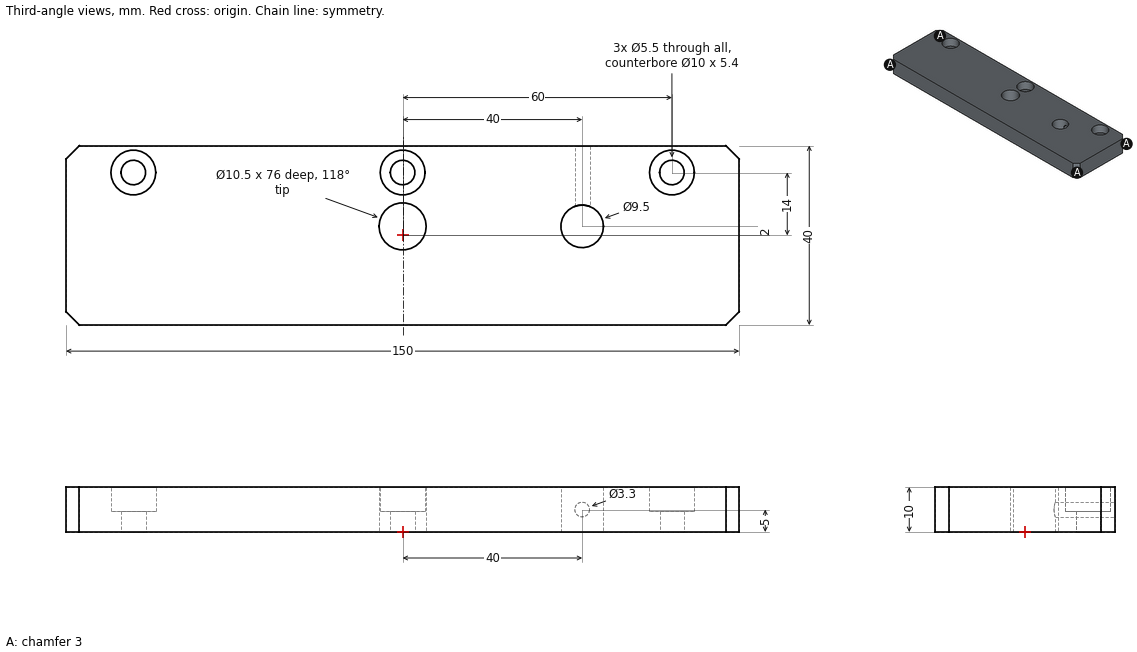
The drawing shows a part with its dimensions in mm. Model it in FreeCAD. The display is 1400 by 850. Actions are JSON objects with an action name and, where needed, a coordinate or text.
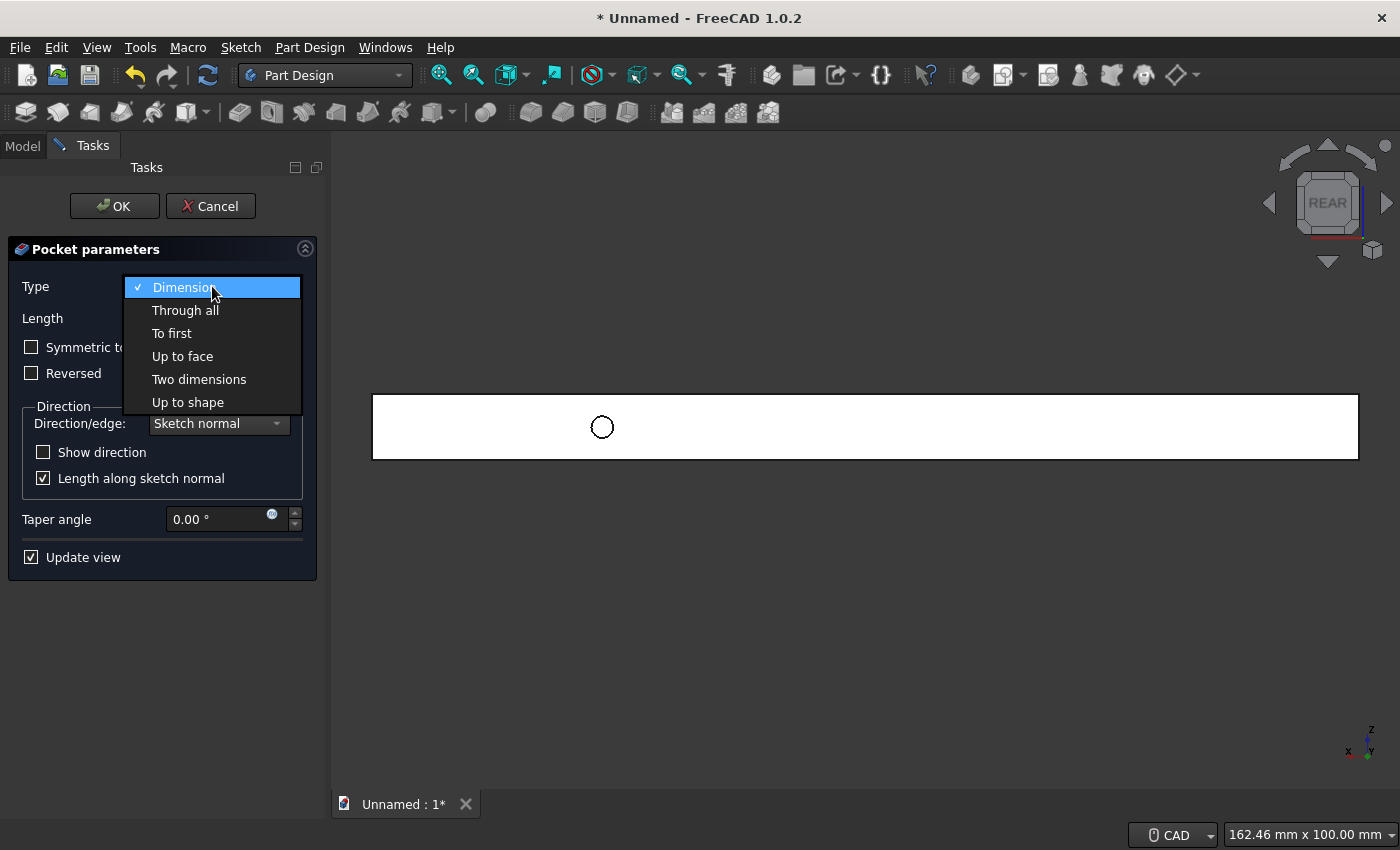
{"action": "left_click", "coordinate": [212, 334]}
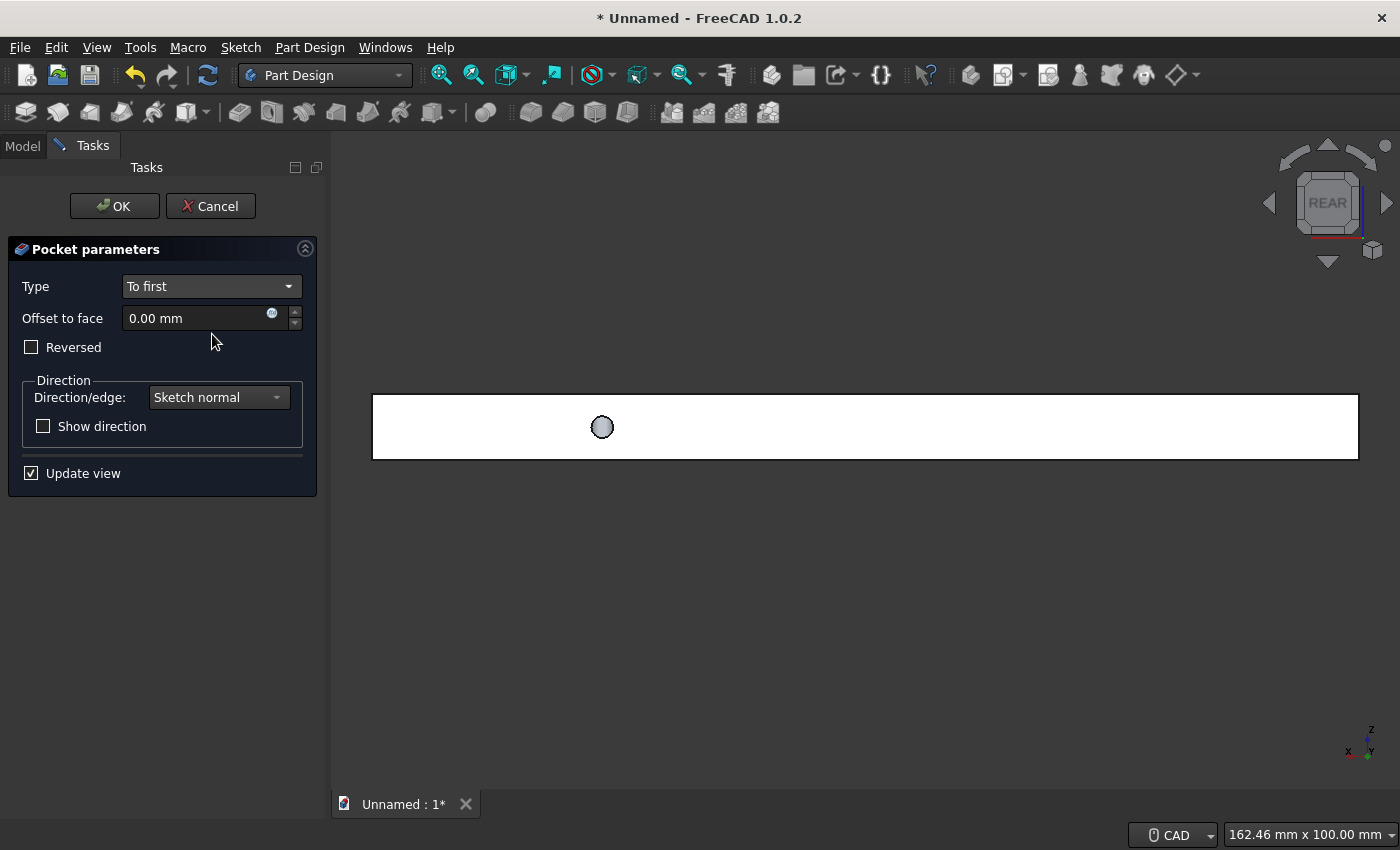
{"action": "left_click", "coordinate": [115, 206]}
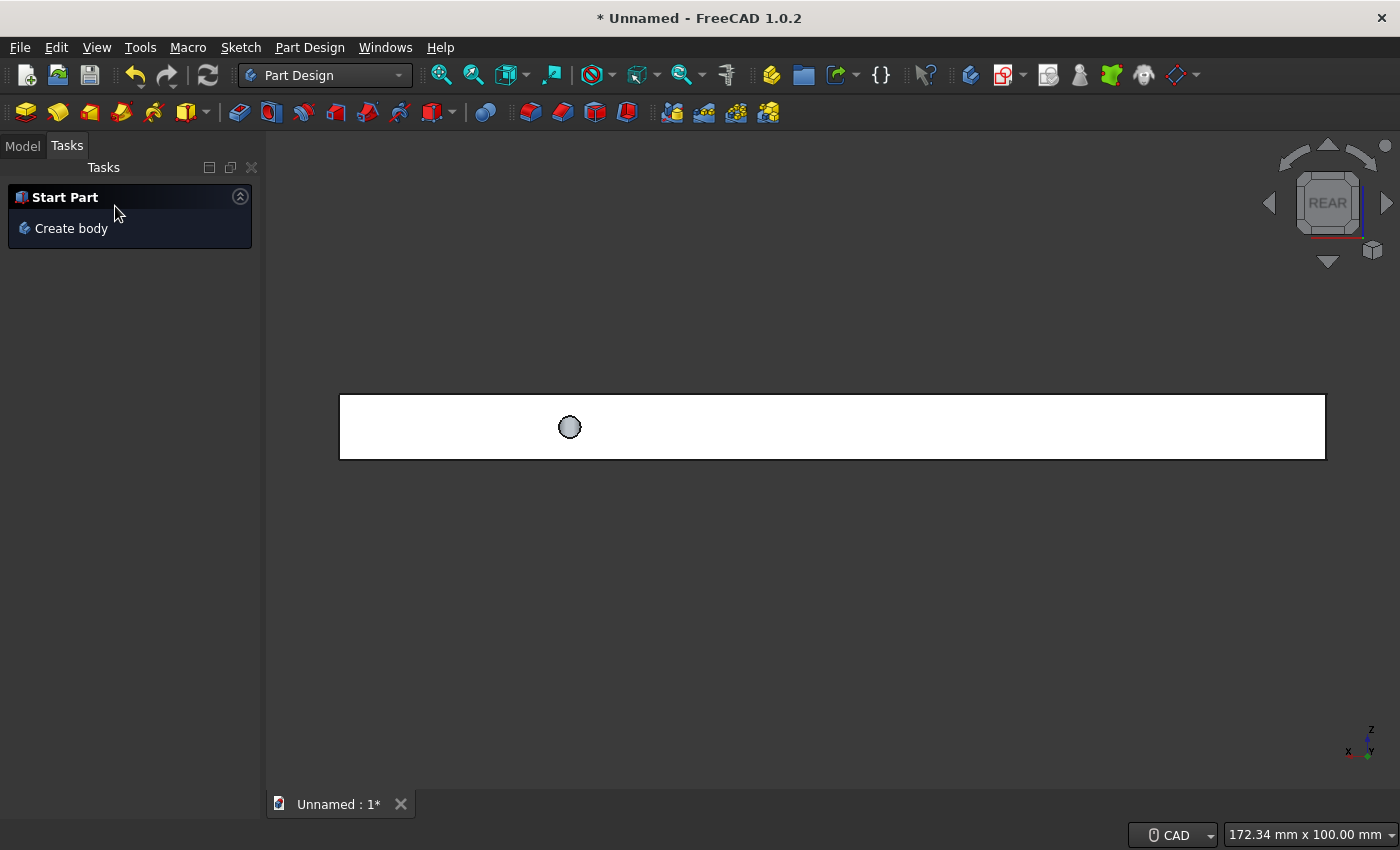
{"action": "left_click", "coordinate": [1327, 426]}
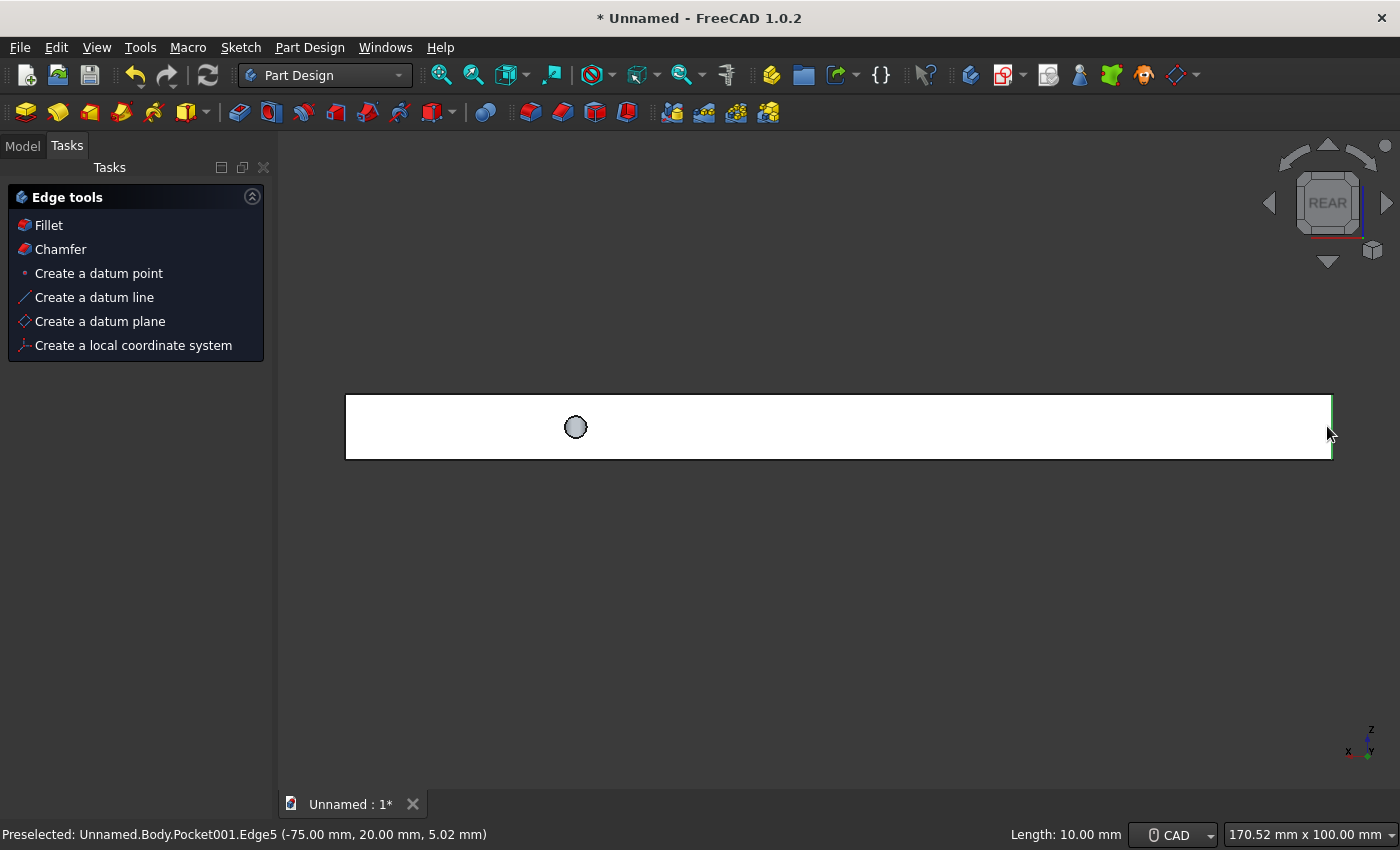
{"action": "key", "text": "0"}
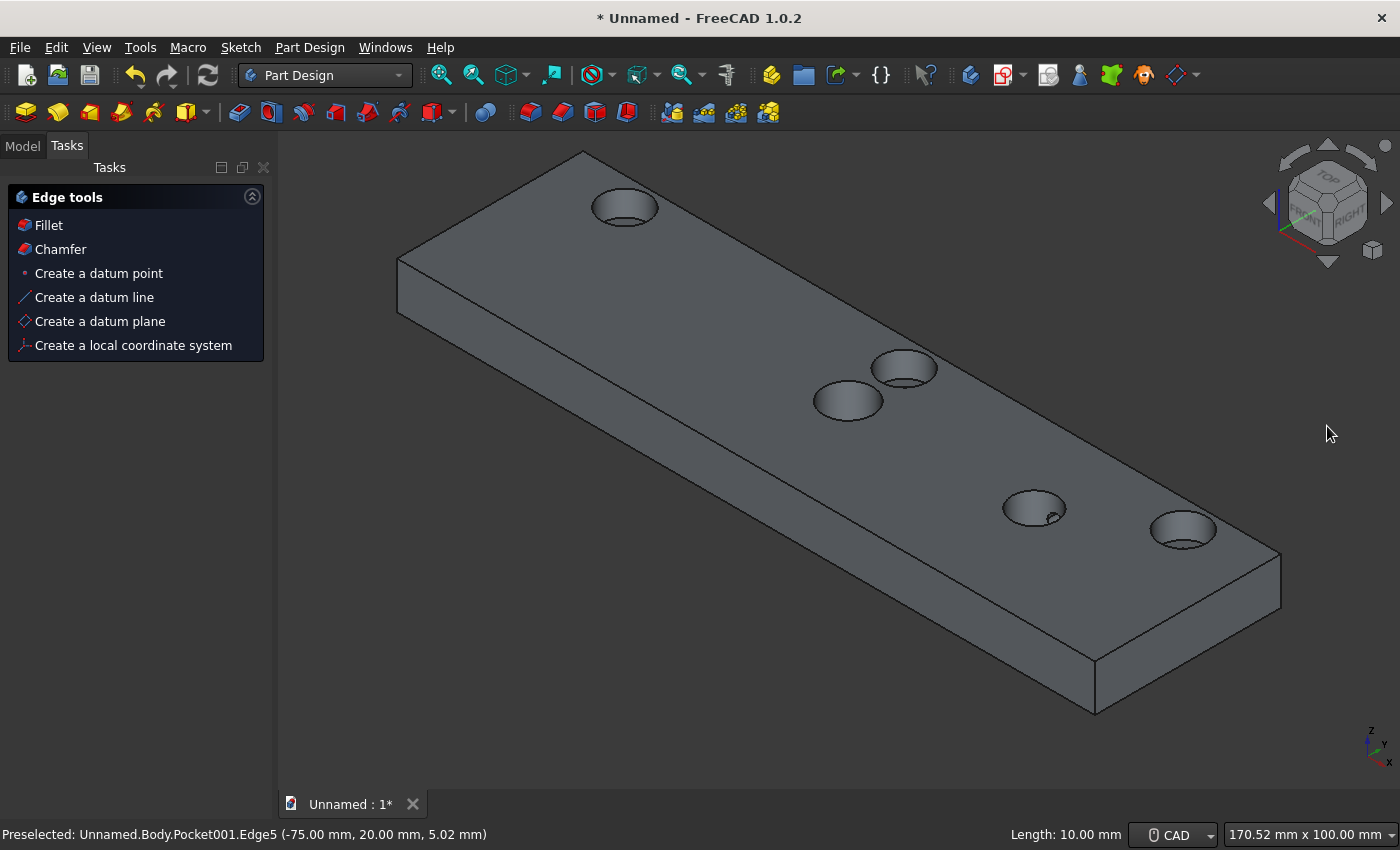
{"action": "left_click", "coordinate": [1095, 687], "text": "ctrl"}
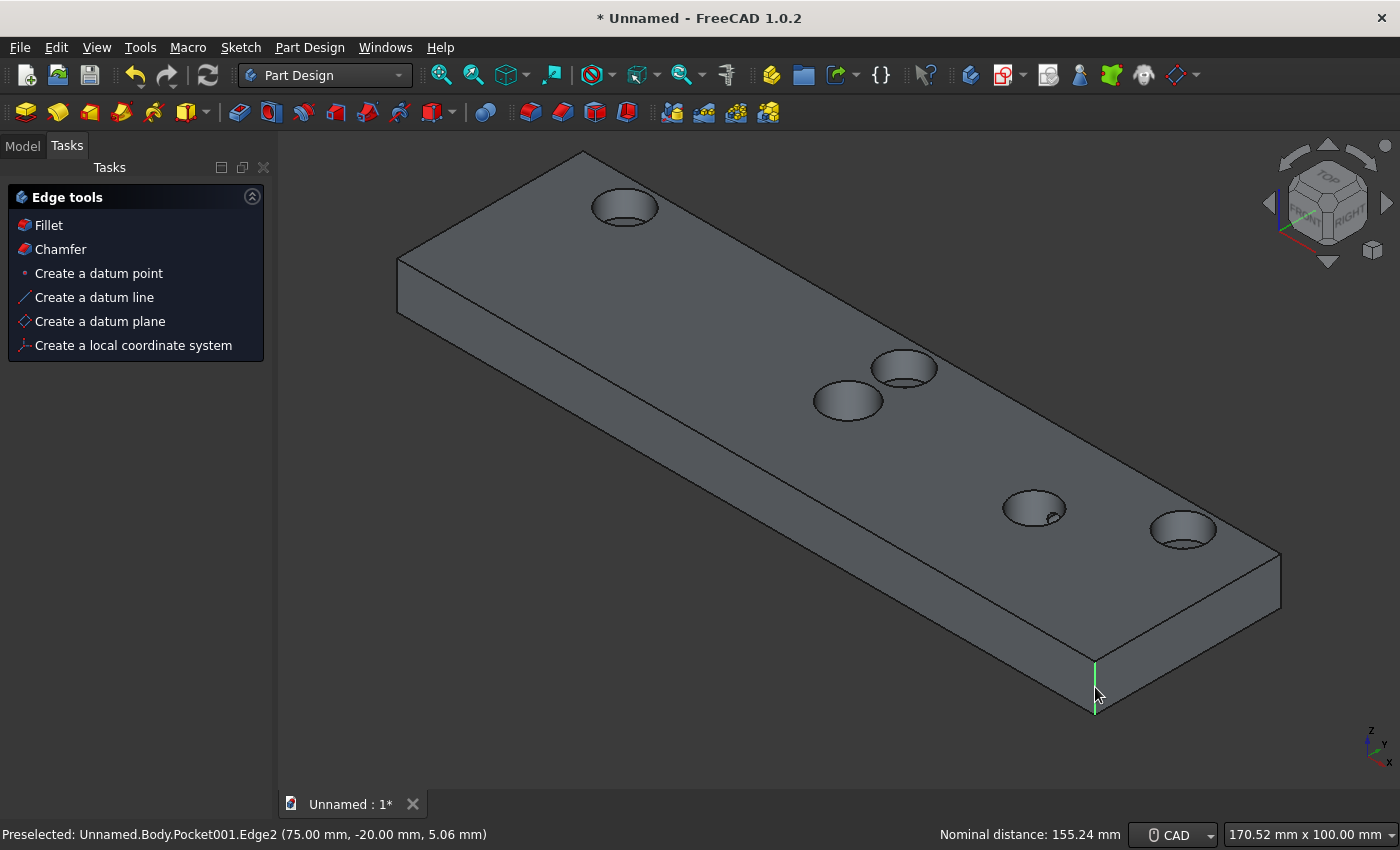
{"action": "key", "text": "2"}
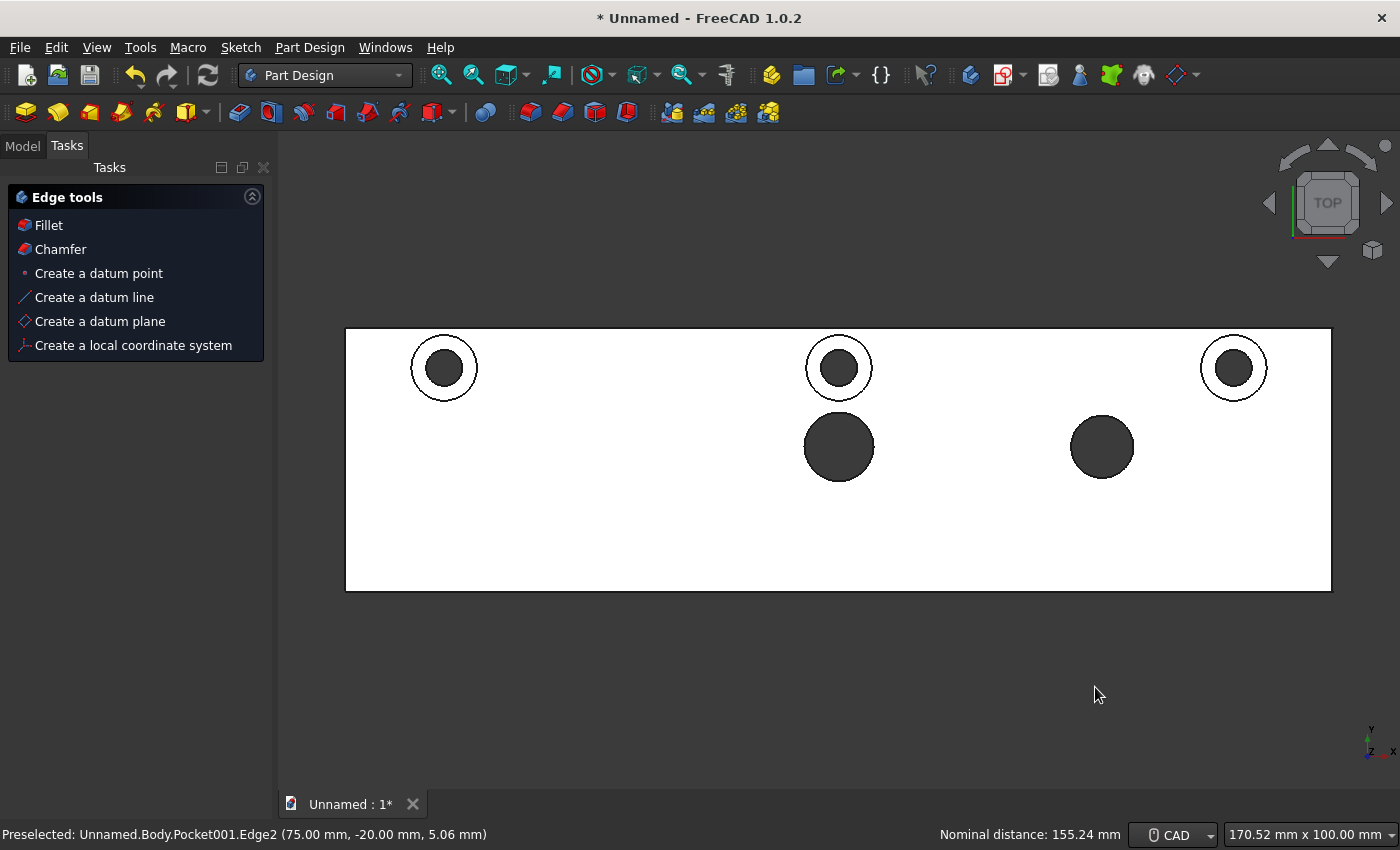
{"action": "key", "text": "1"}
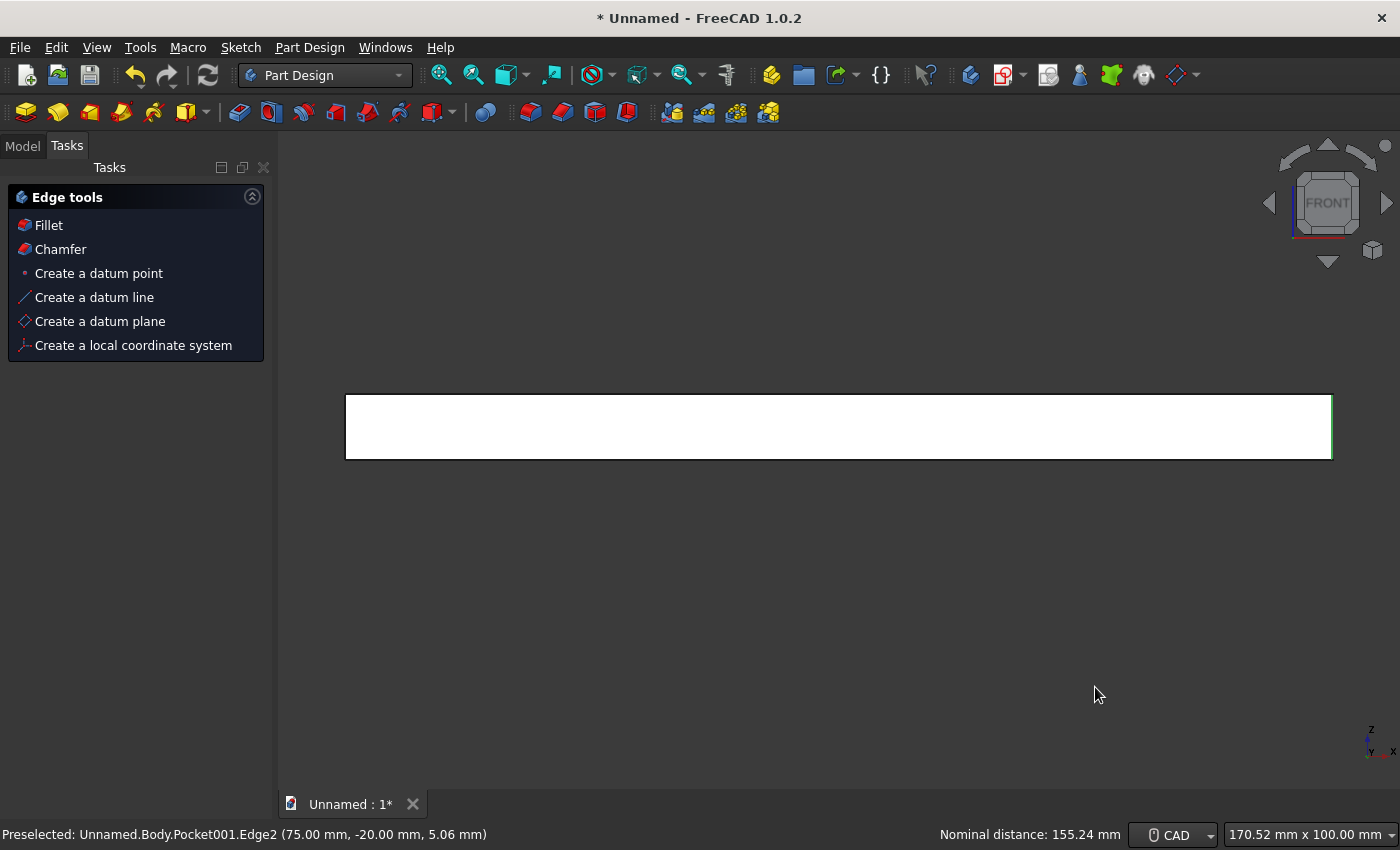
{"action": "left_click", "coordinate": [345, 426], "text": "ctrl"}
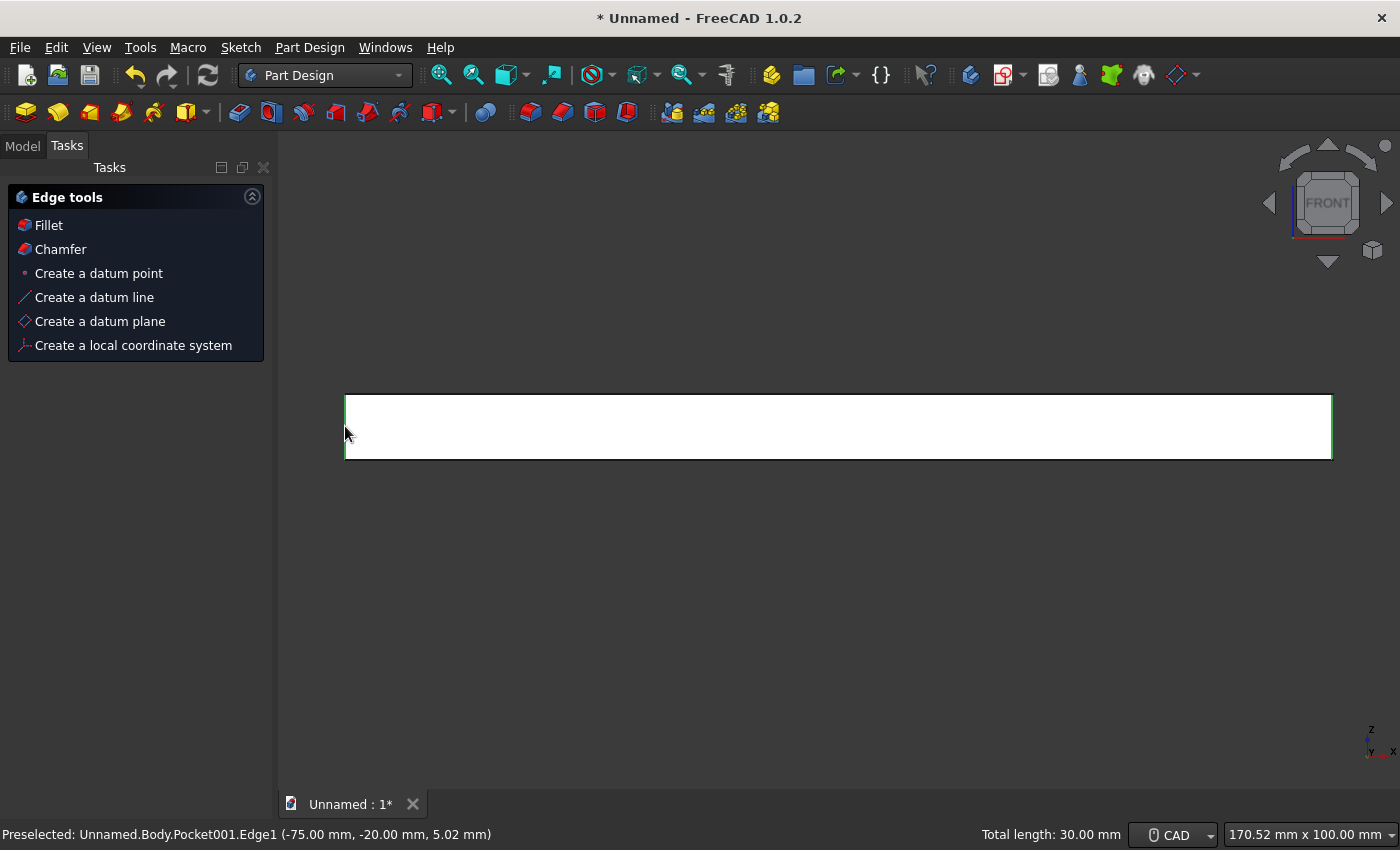
{"action": "key", "text": "3"}